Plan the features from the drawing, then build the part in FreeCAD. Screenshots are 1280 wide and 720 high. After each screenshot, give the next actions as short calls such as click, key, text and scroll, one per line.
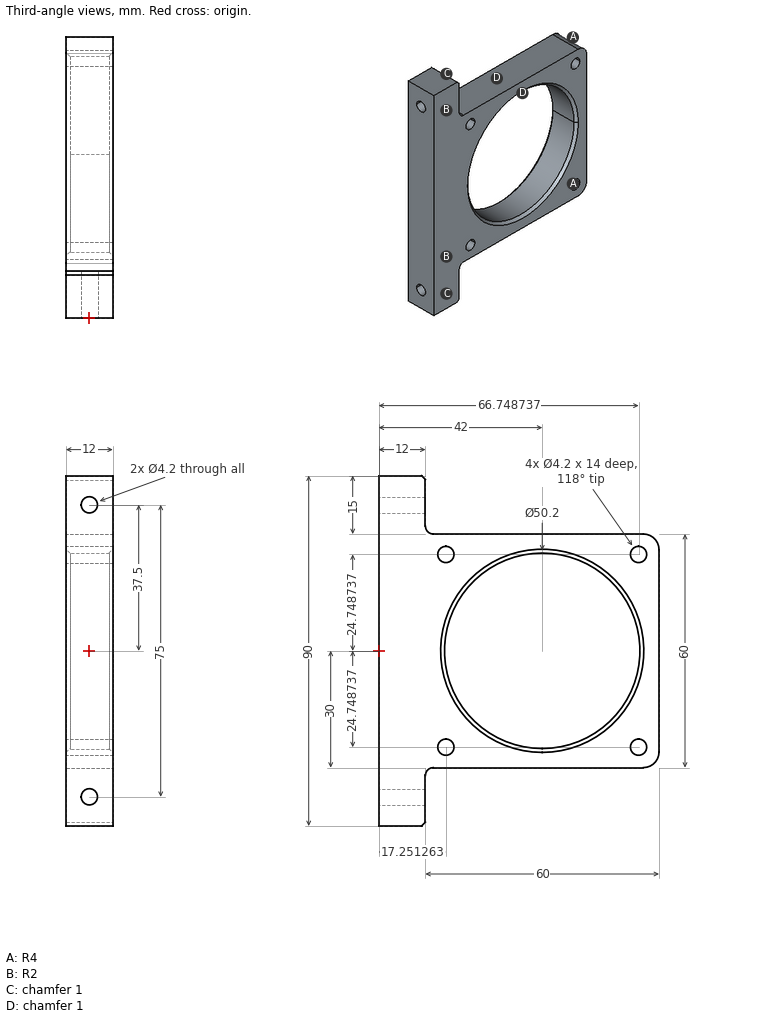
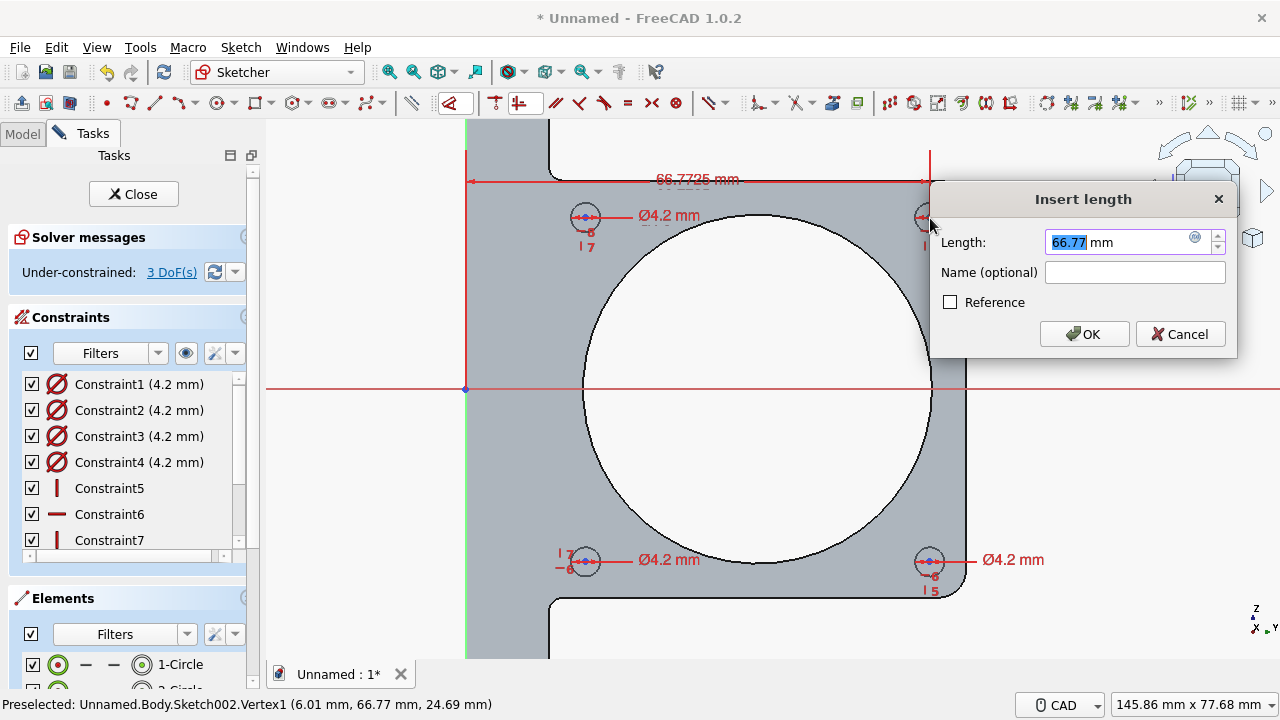
text(66.748737)
key(Return)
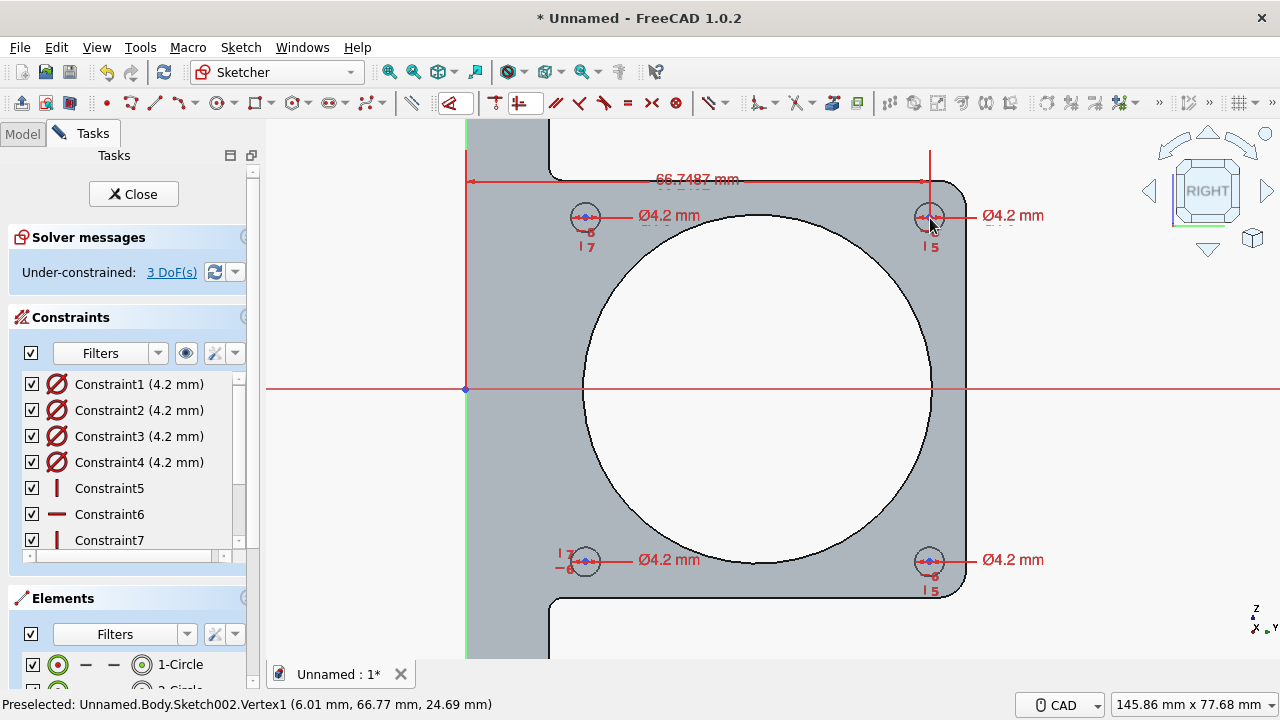
click(930, 218)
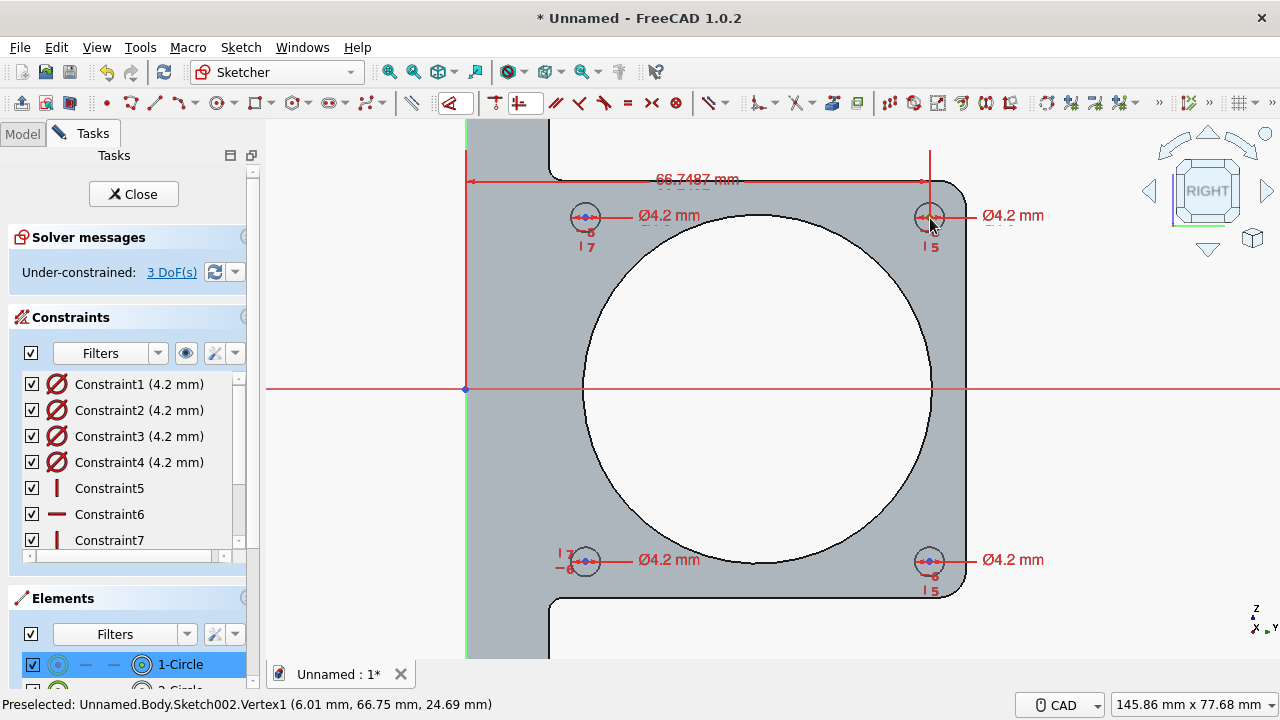
click(468, 104)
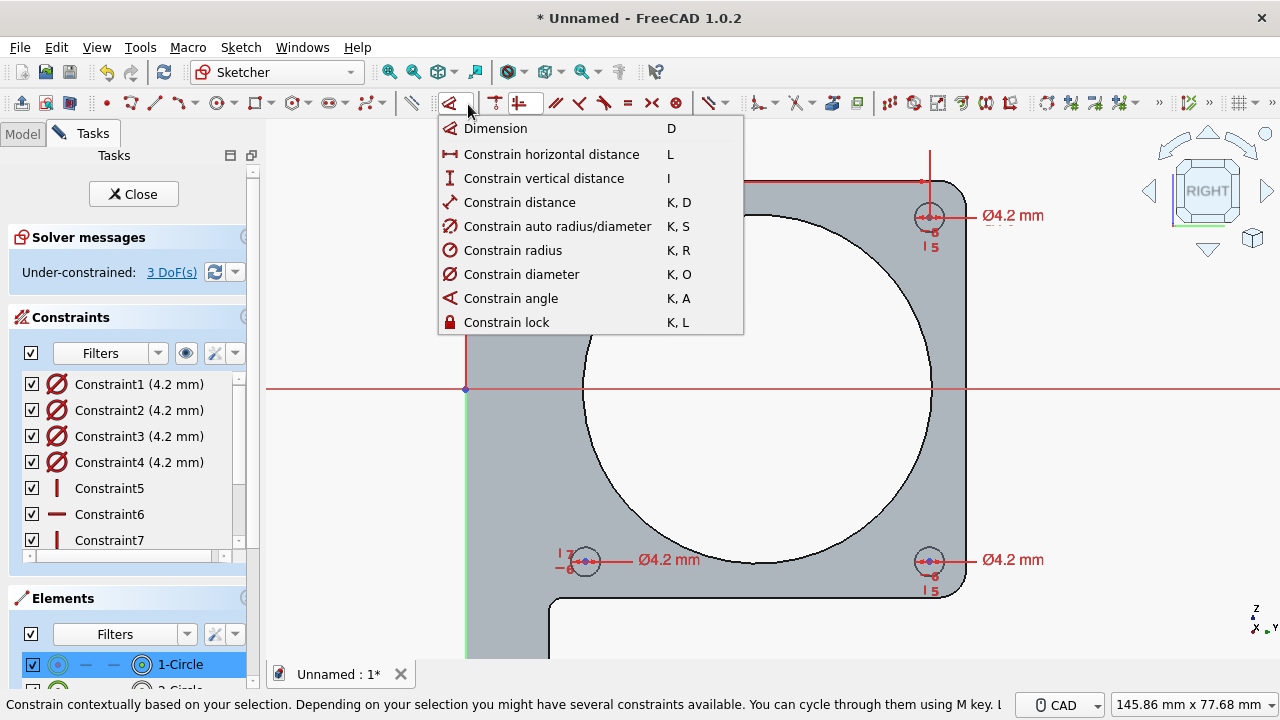
click(591, 178)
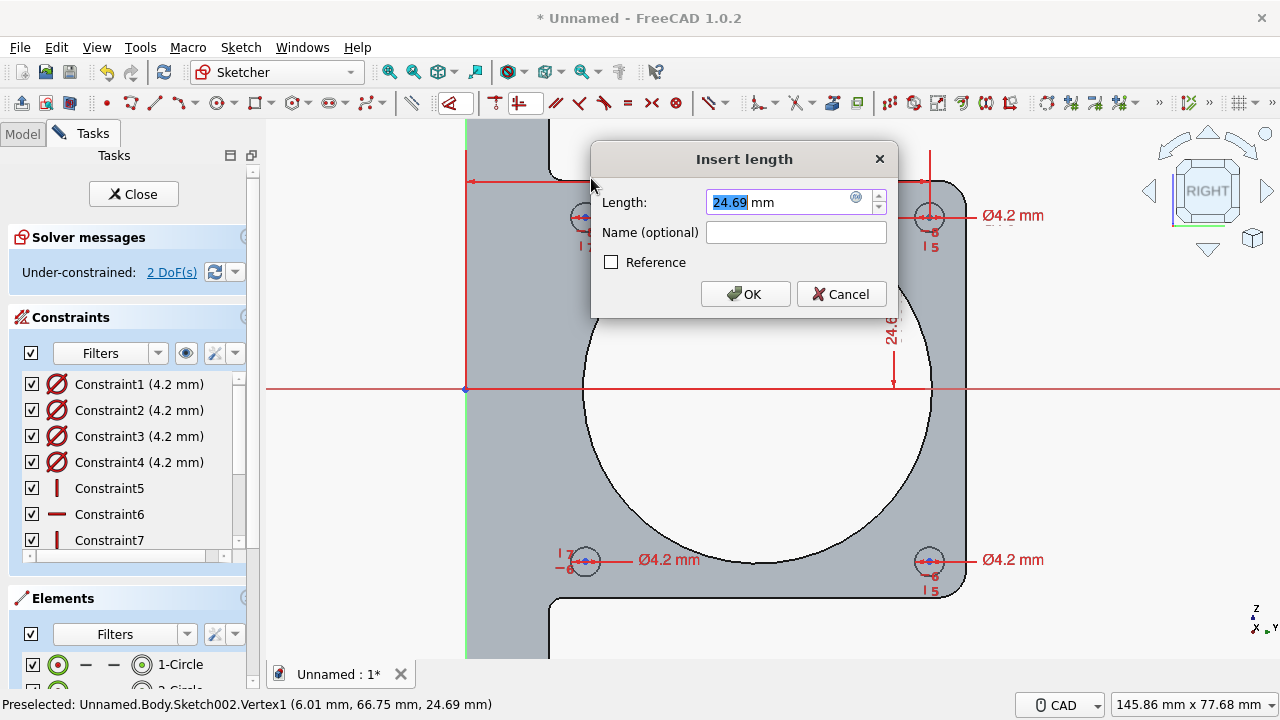
text(24.748737)
key(Return)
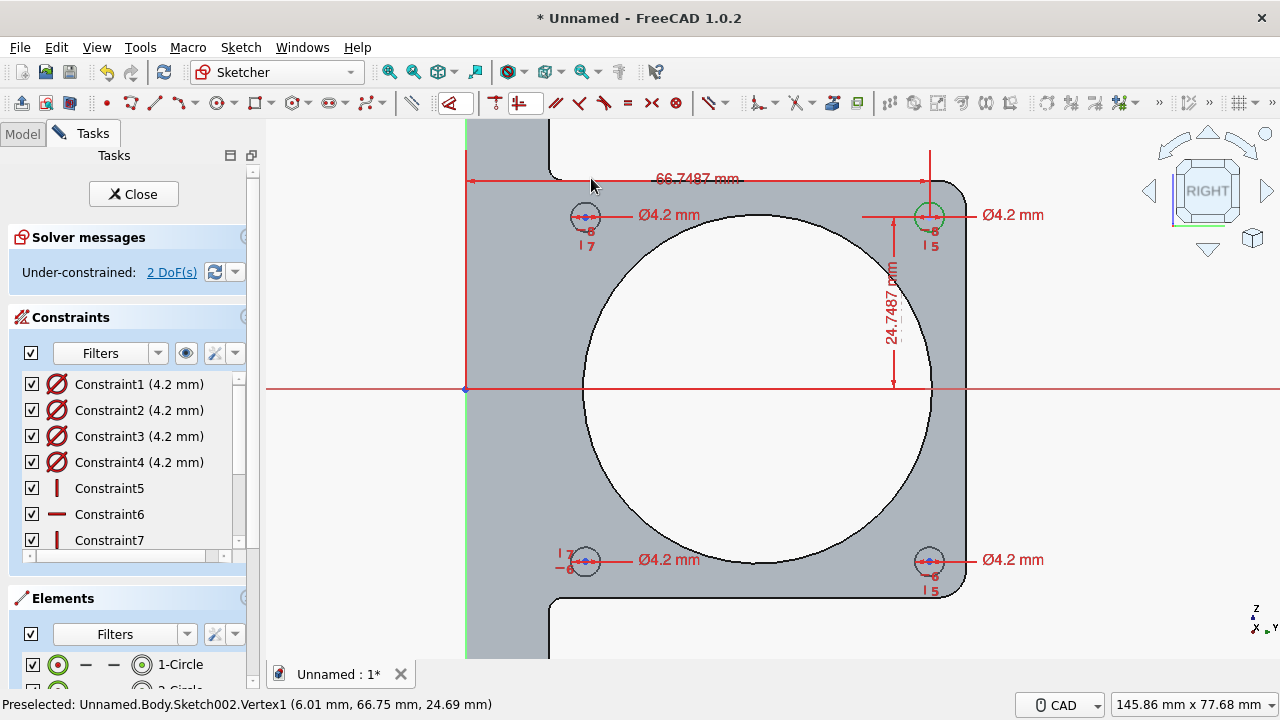
click(930, 562)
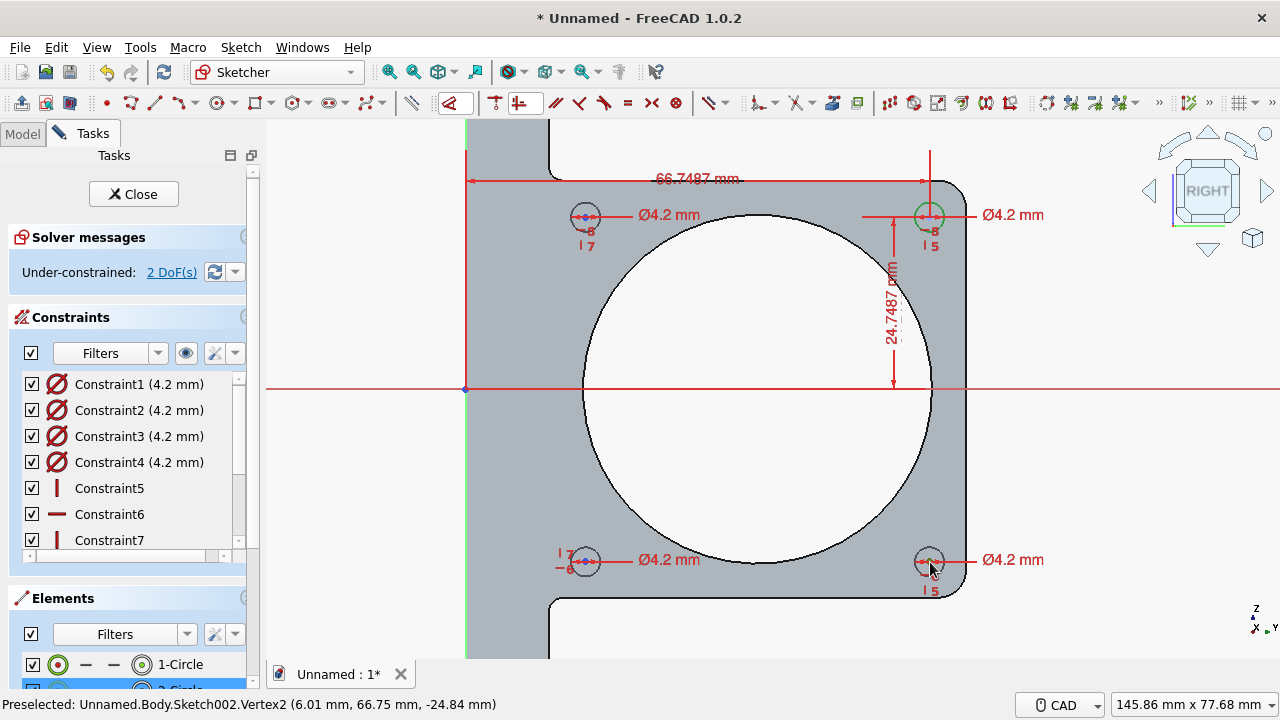
click(468, 104)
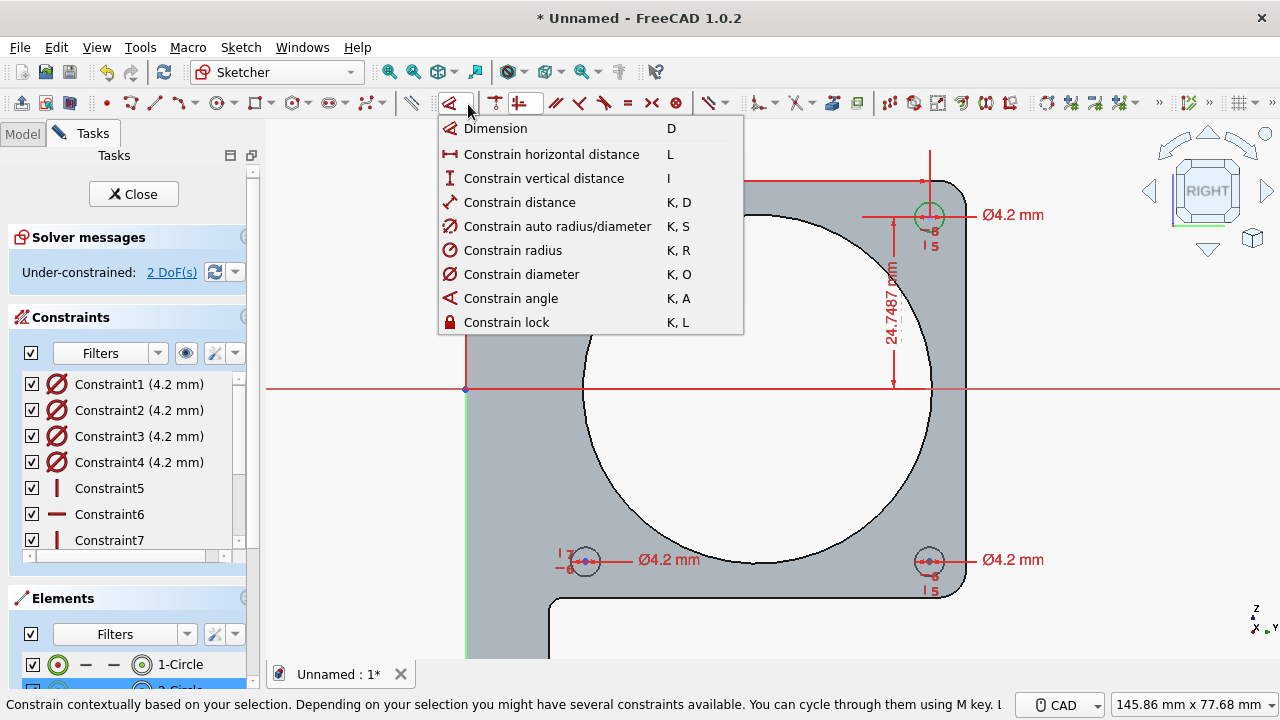
click(591, 178)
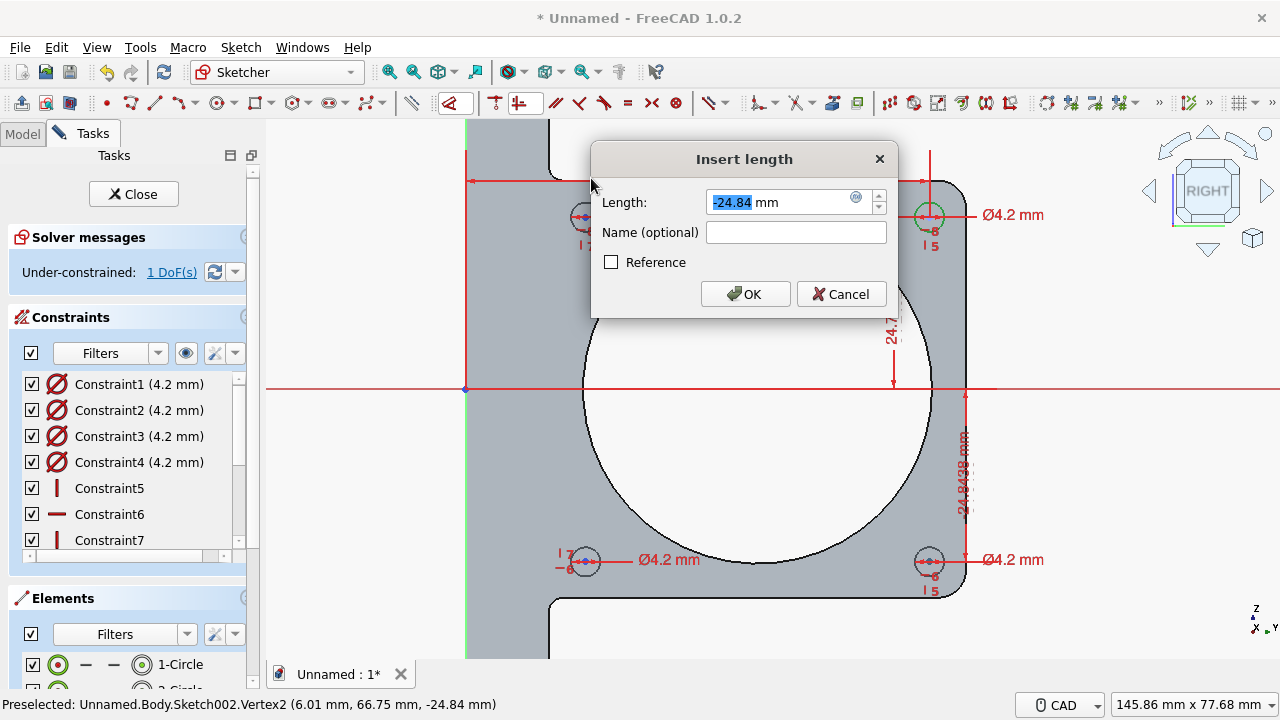
text(-24.748737)
key(Return)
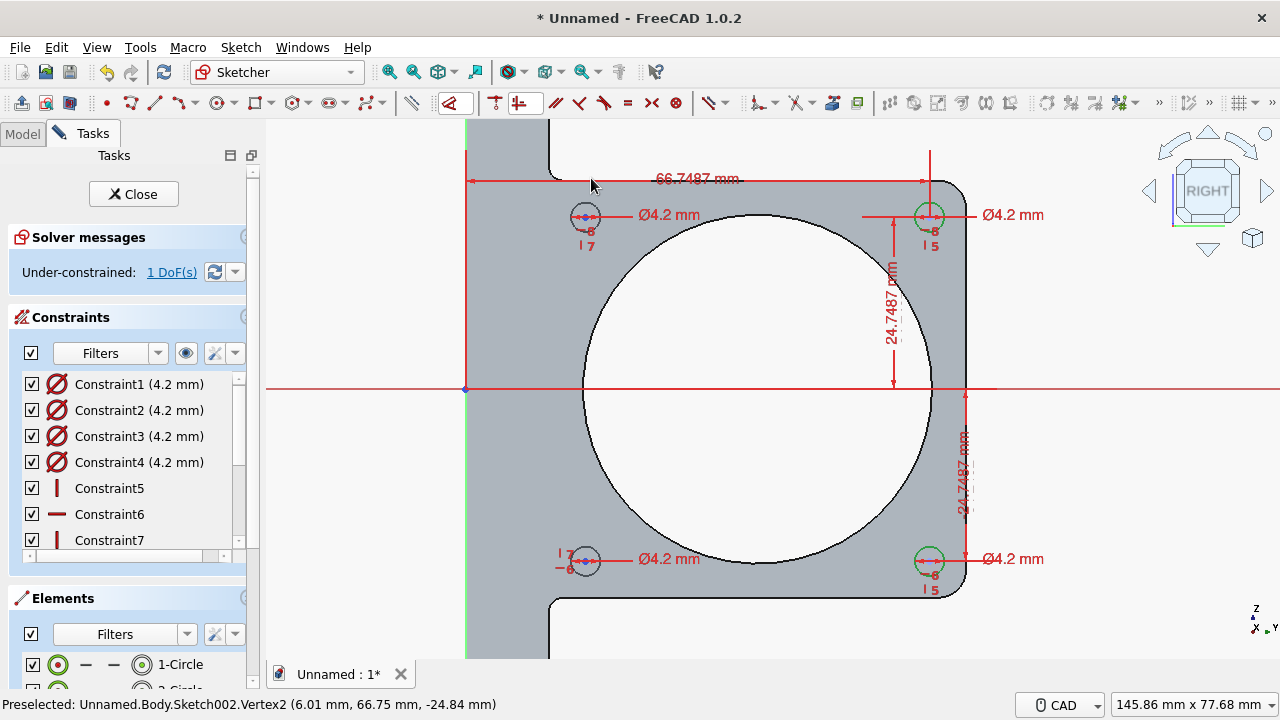
click(586, 561)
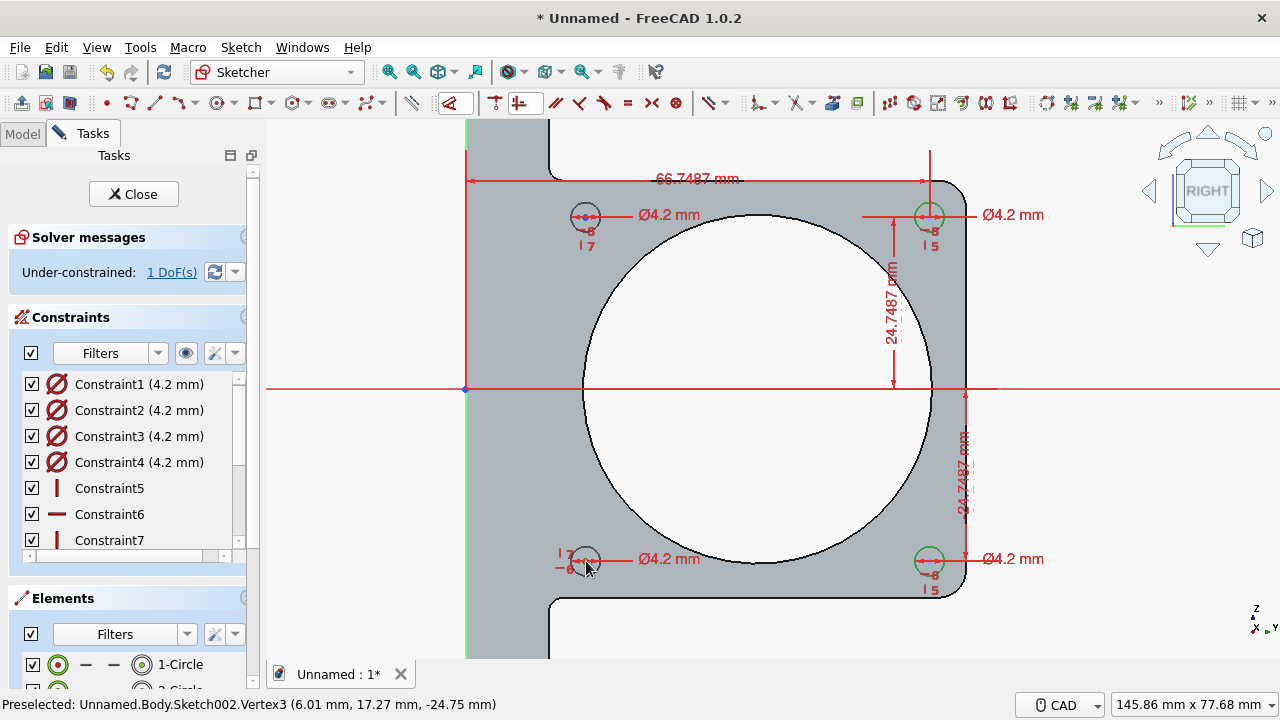
key(l)